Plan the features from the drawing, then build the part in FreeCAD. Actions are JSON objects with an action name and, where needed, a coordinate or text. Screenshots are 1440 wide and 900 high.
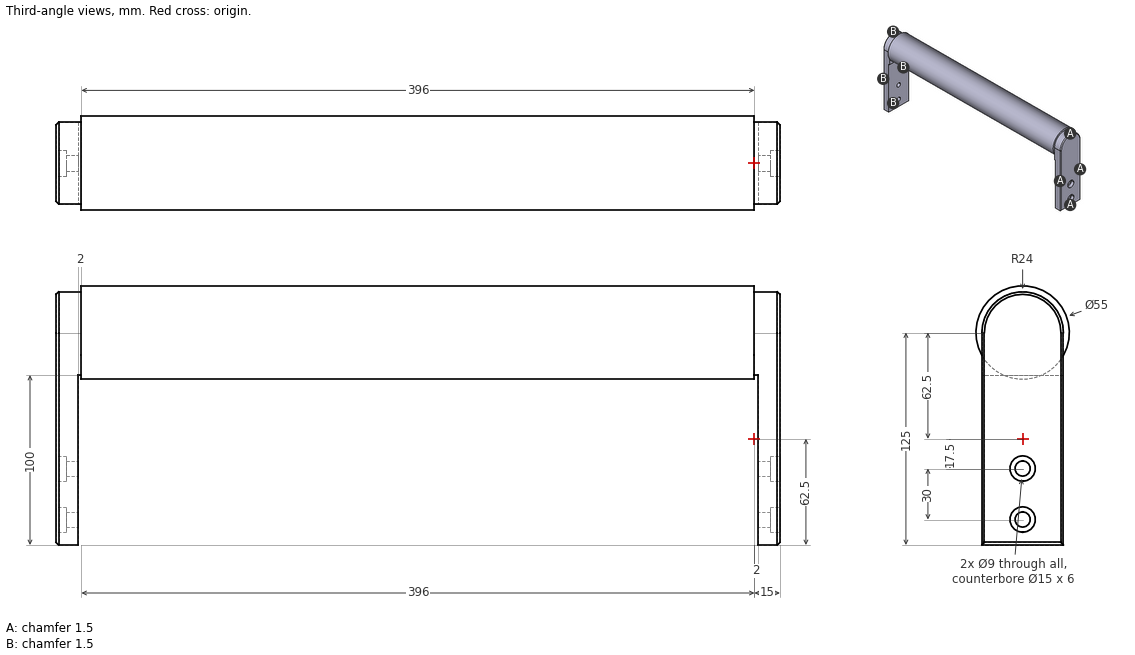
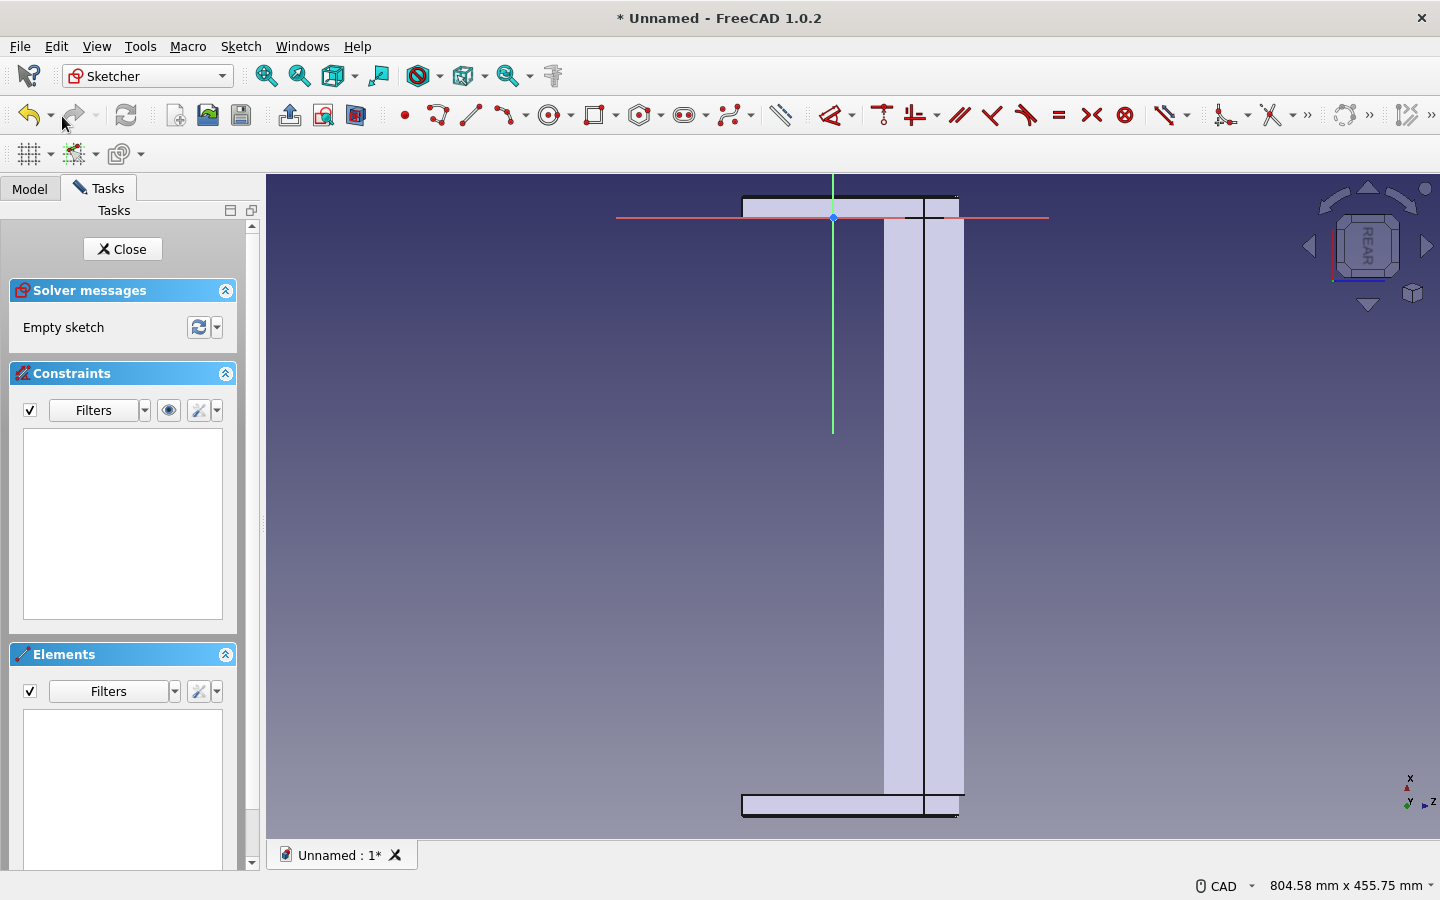
{"action": "left_click", "coordinate": [356, 116]}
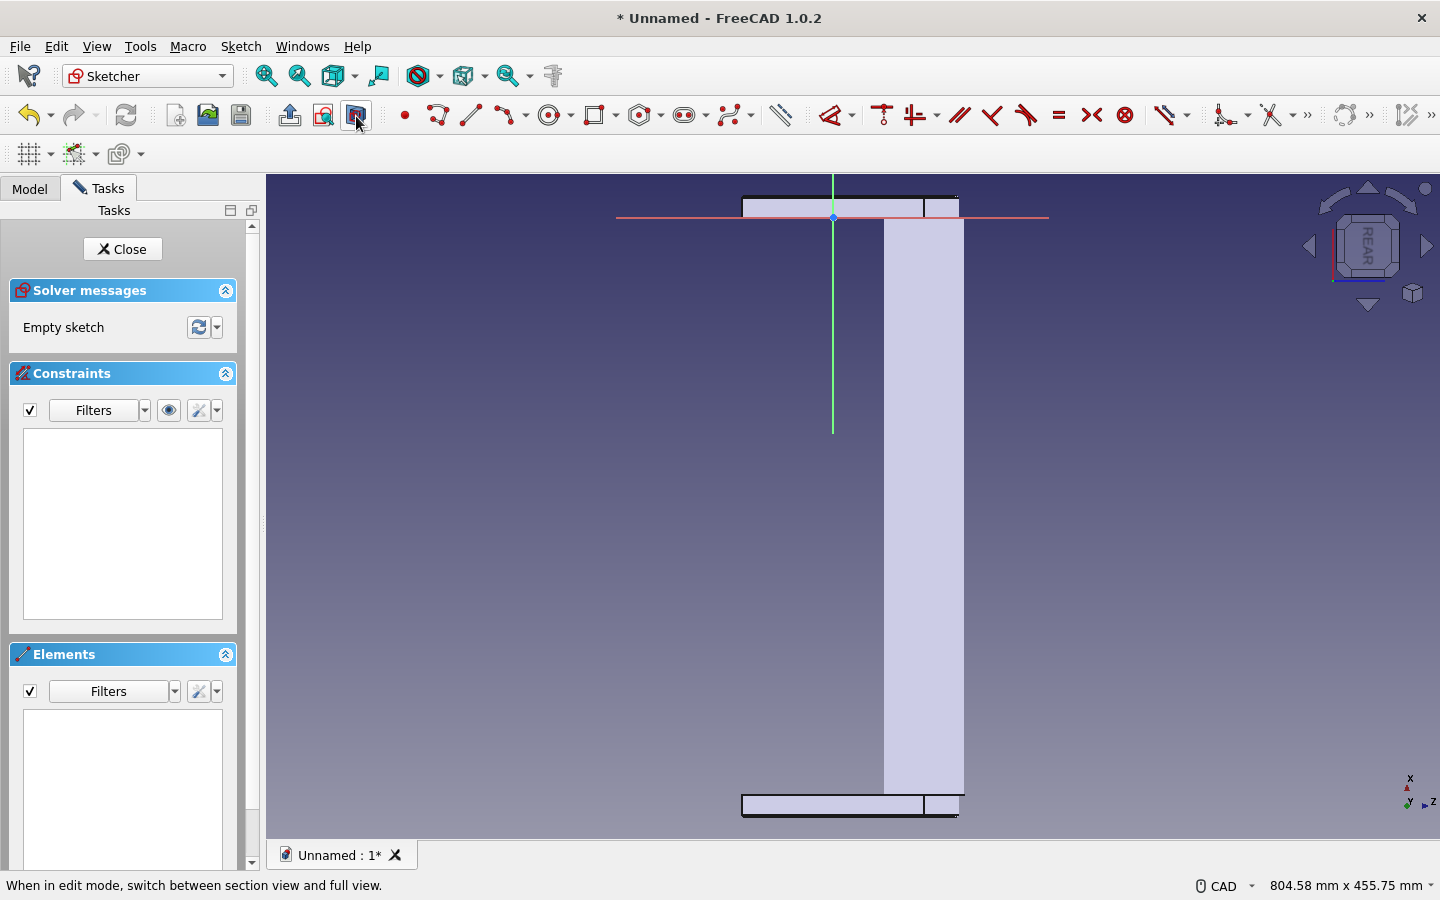
{"action": "scroll", "coordinate": [723, 507], "scroll_direction": "down", "scroll_amount": 2}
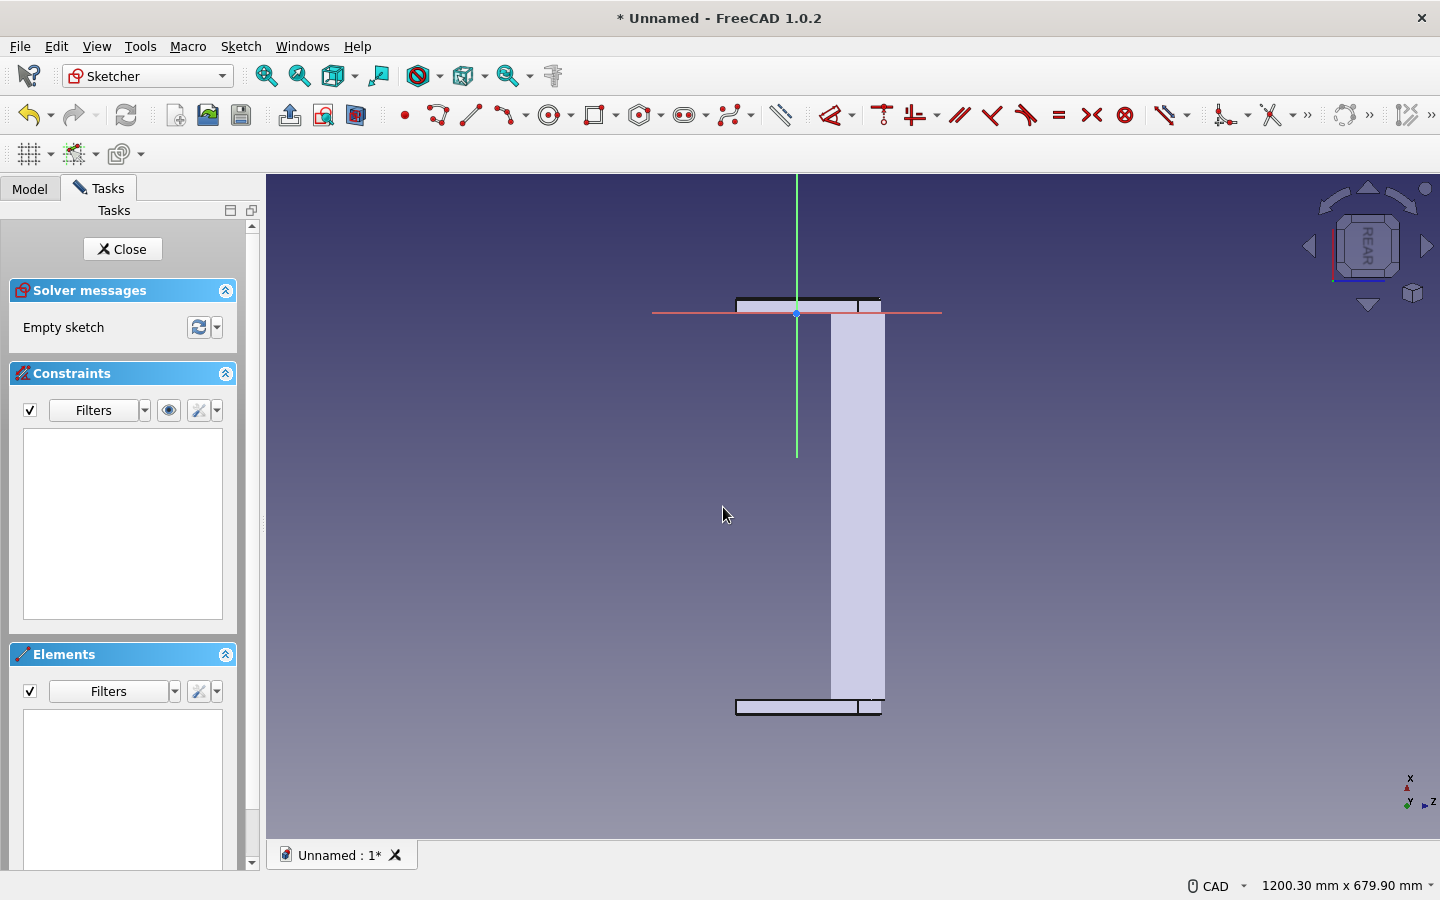
{"action": "left_click", "coordinate": [594, 116]}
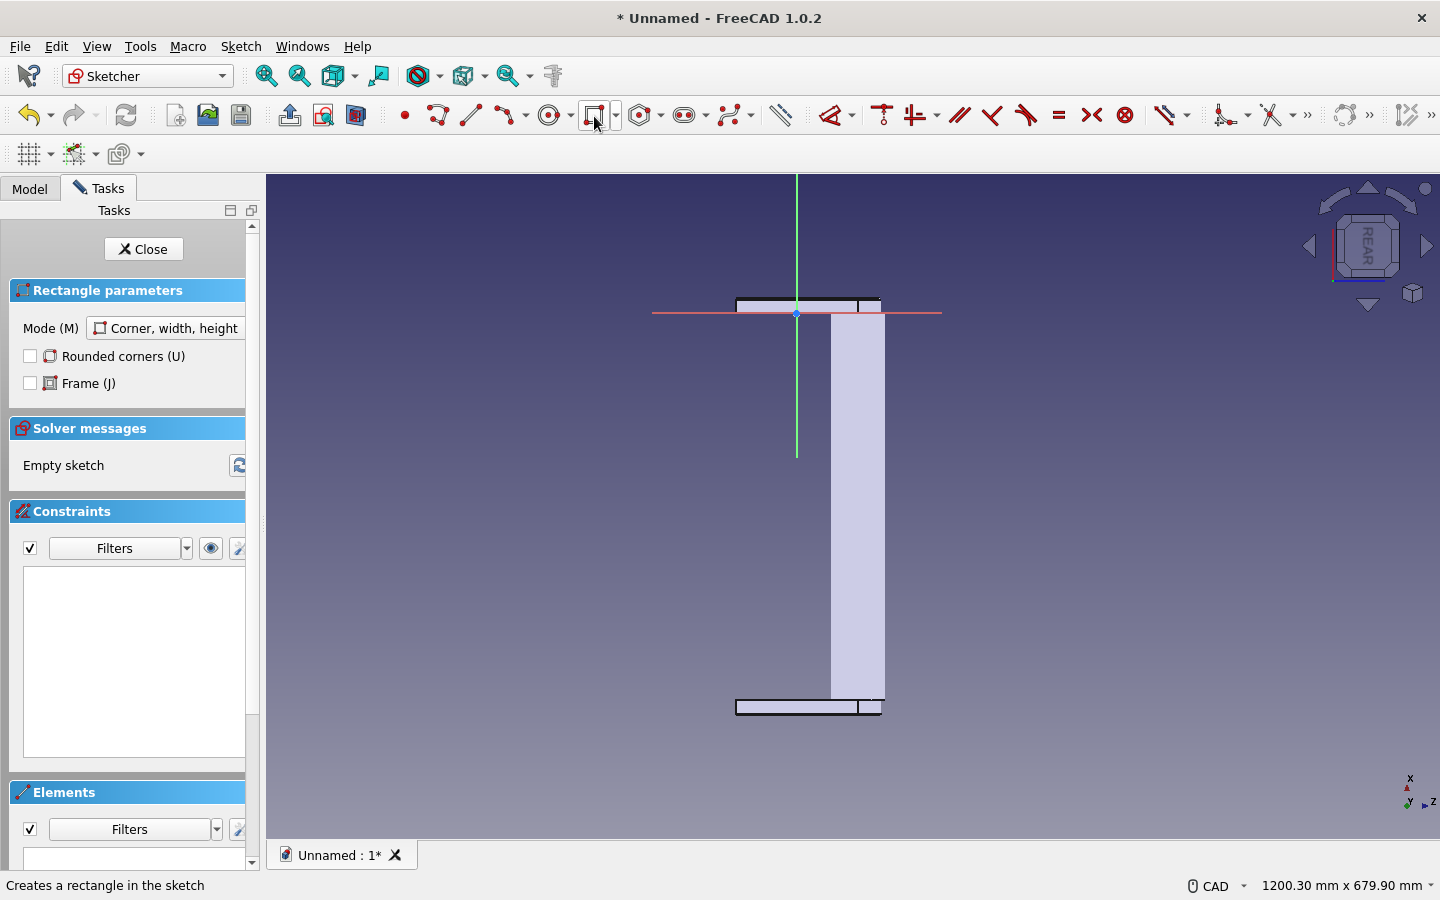
{"action": "scroll", "coordinate": [736, 700], "scroll_direction": "up", "scroll_amount": 11}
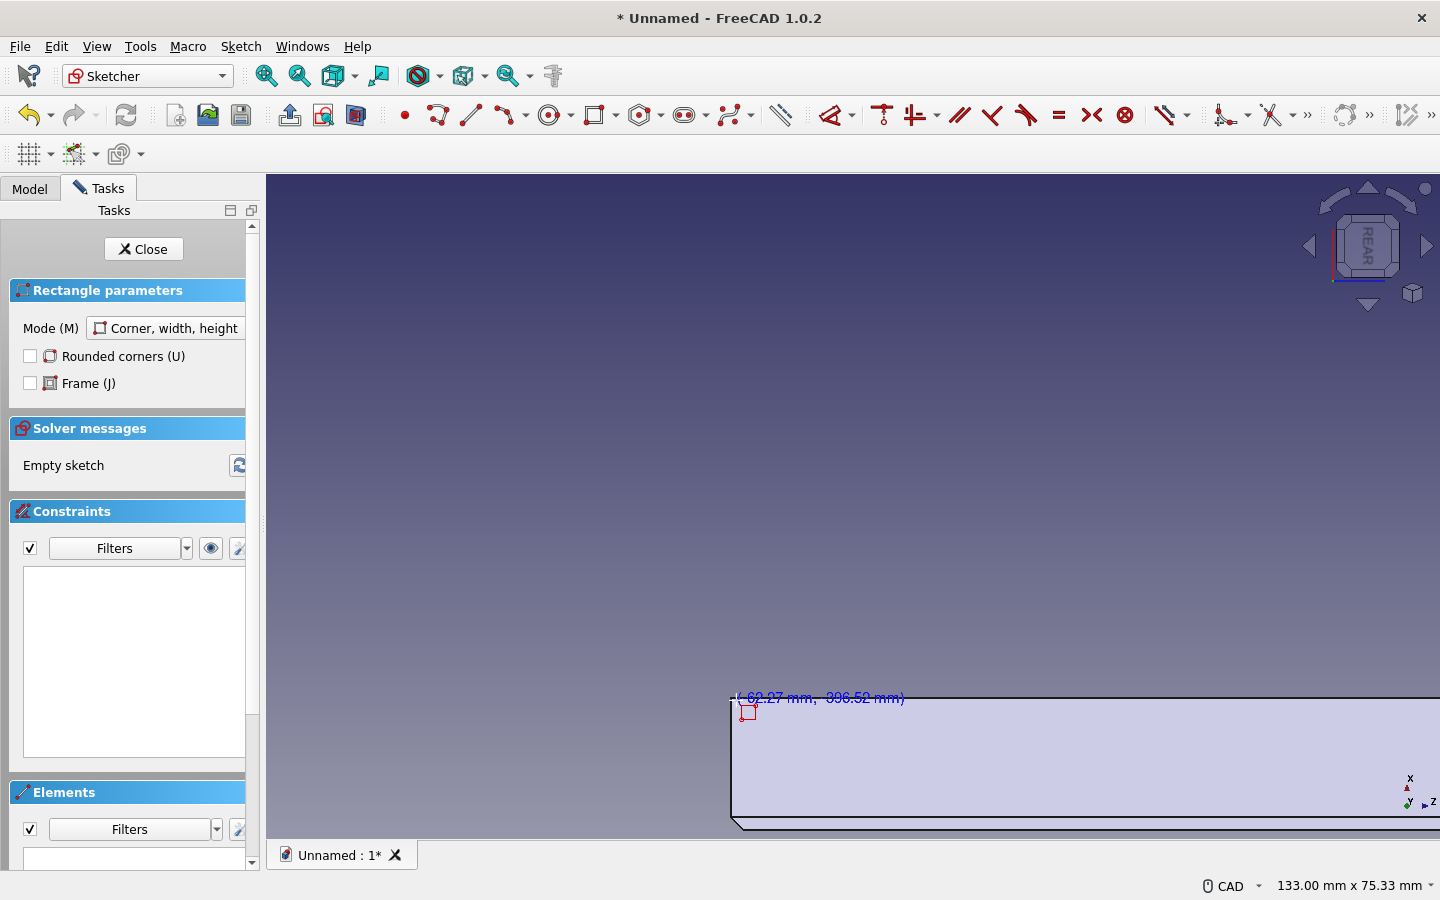
{"action": "scroll", "coordinate": [736, 700], "scroll_direction": "down", "scroll_amount": 11}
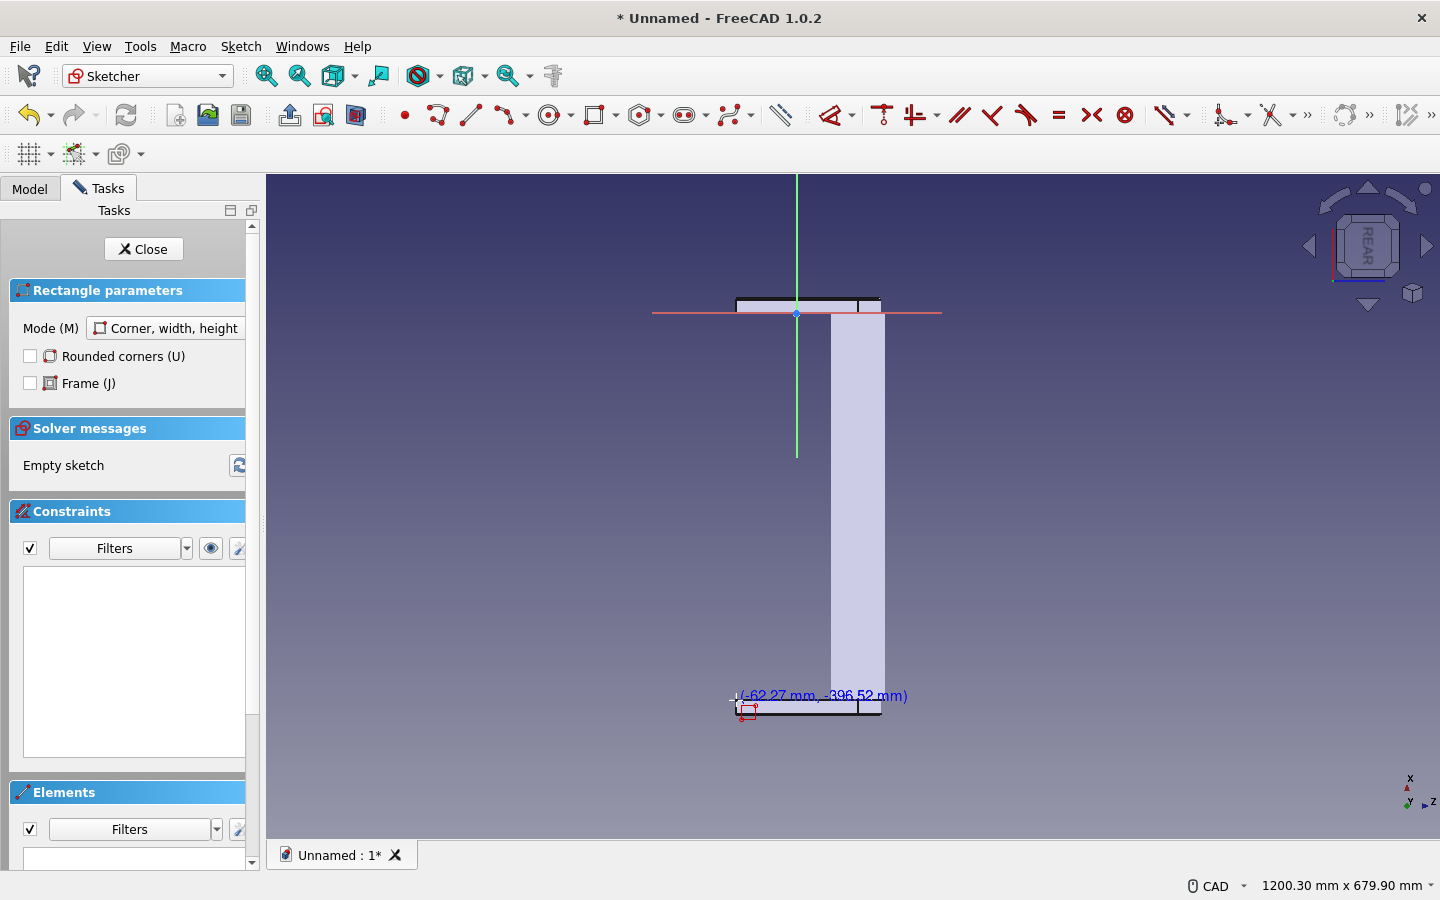
{"action": "left_click", "coordinate": [736, 700]}
{"action": "mouse_move", "coordinate": [834, 702]}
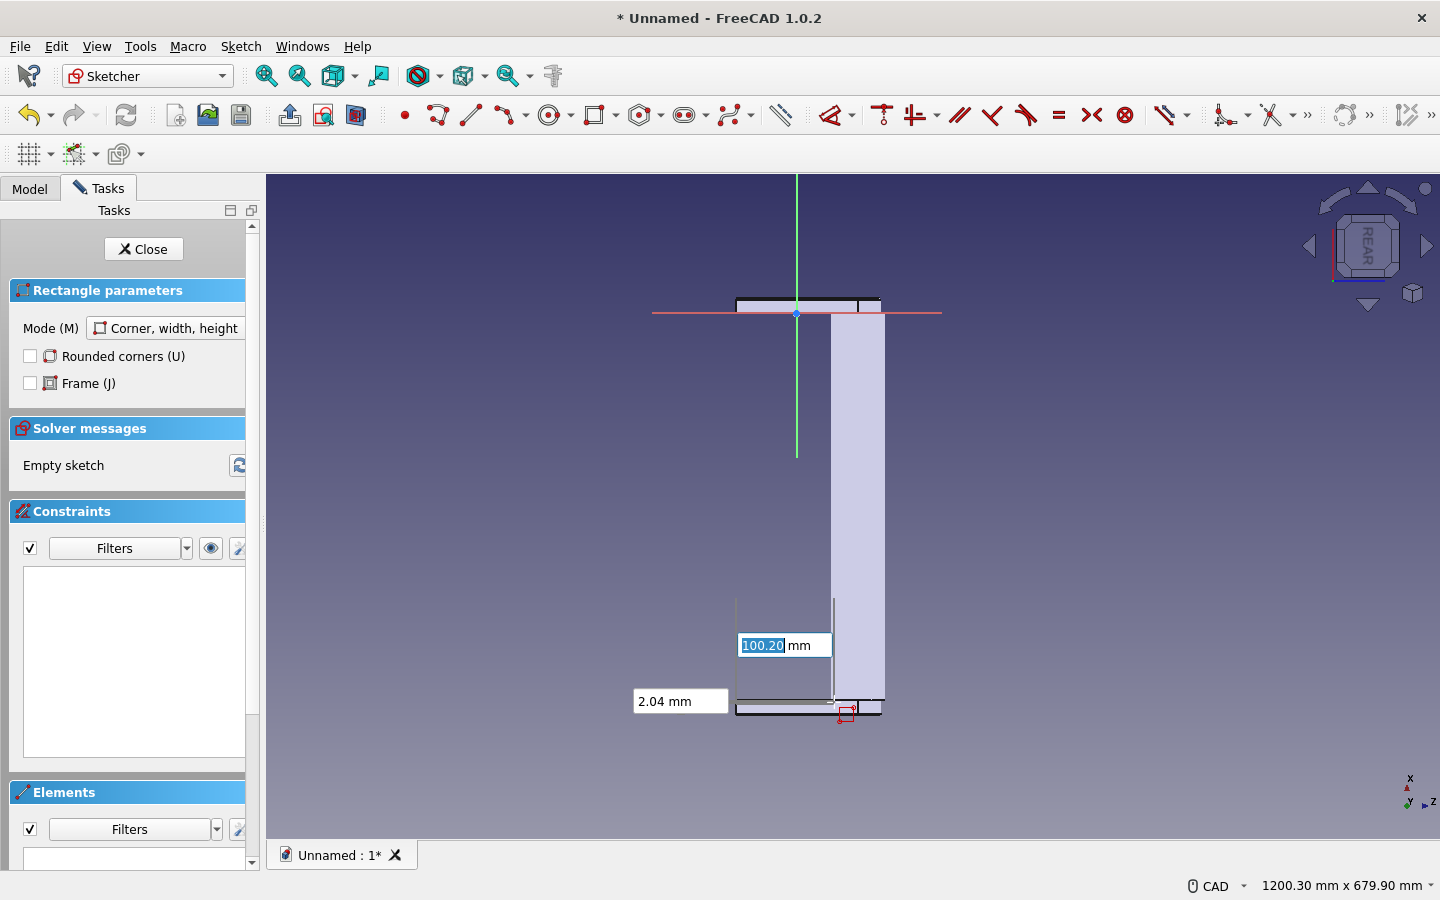
{"action": "type", "text": "100"}
{"action": "key", "text": "Tab"}
{"action": "type", "text": "2"}
{"action": "key", "text": "Return"}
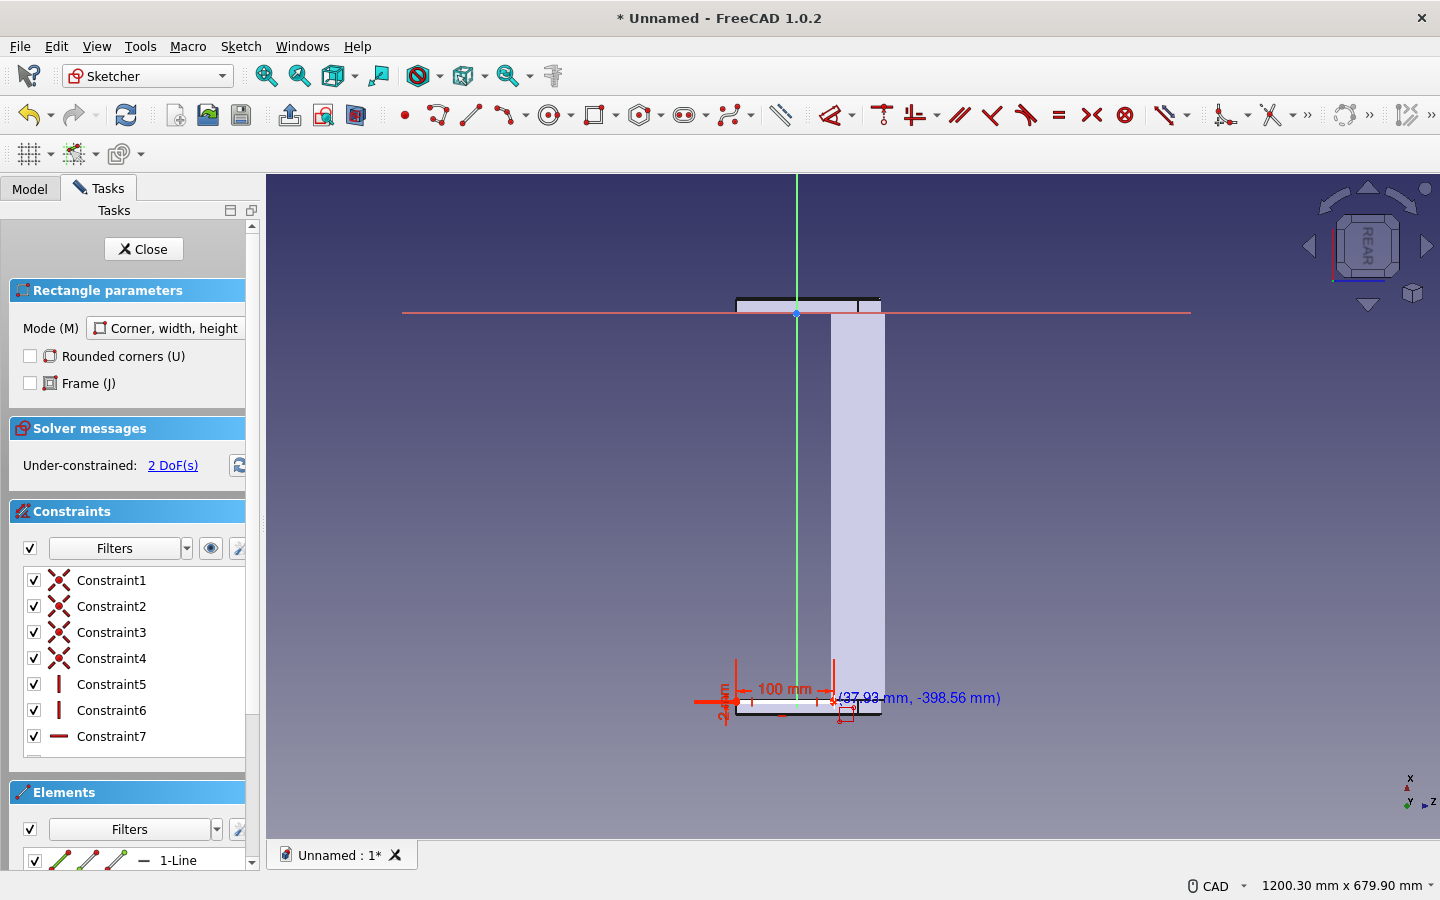
{"action": "scroll", "coordinate": [736, 311], "scroll_direction": "up", "scroll_amount": 11}